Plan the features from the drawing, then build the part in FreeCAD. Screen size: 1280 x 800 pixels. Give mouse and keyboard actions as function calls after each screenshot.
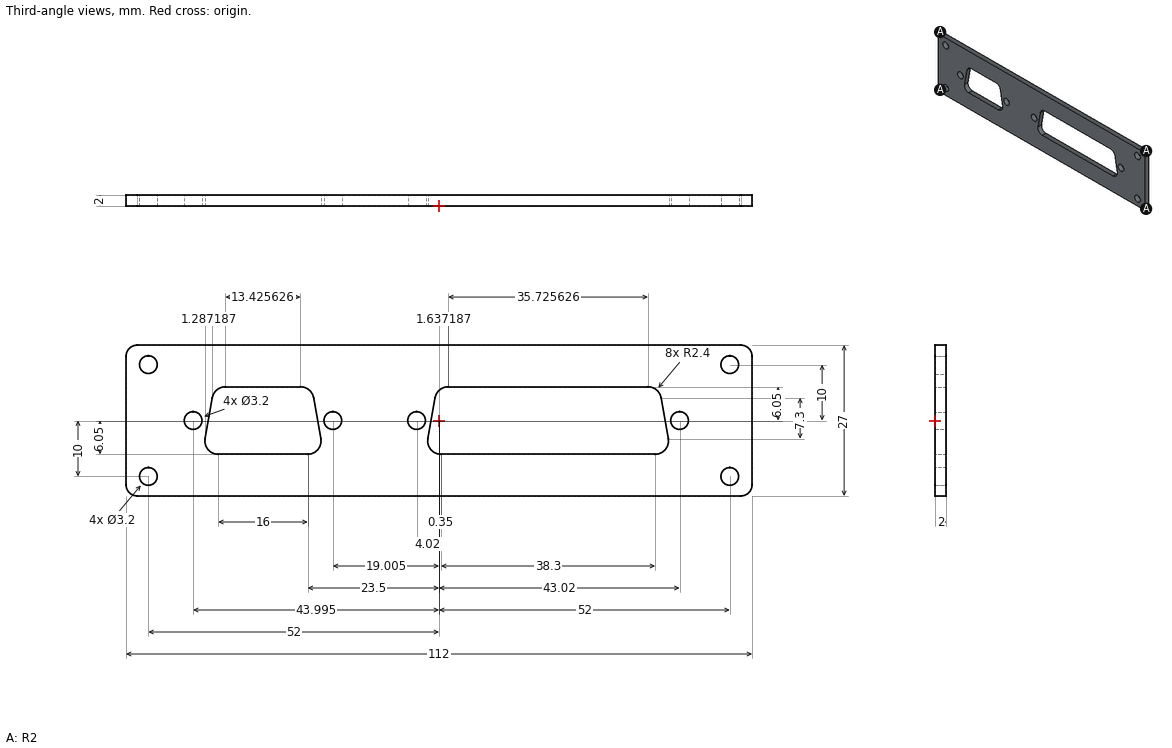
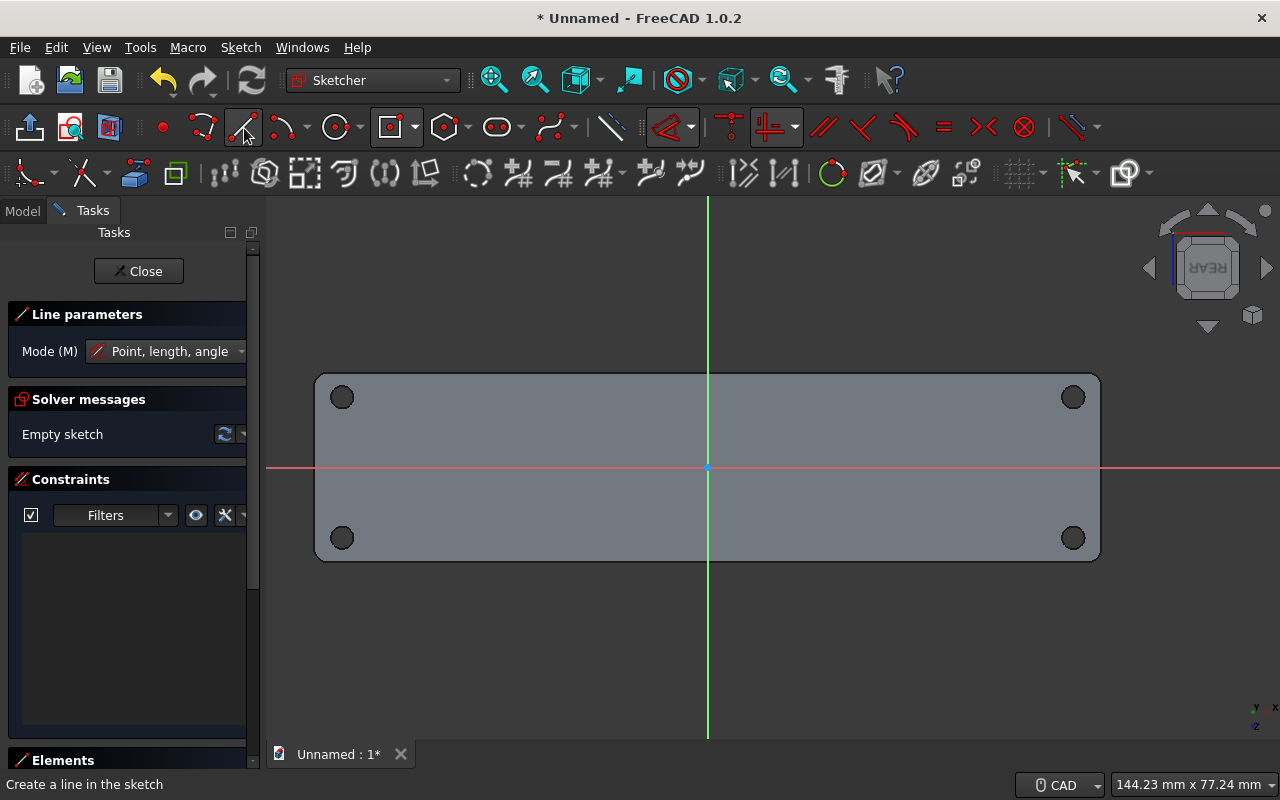
scroll(719, 510, up, 2)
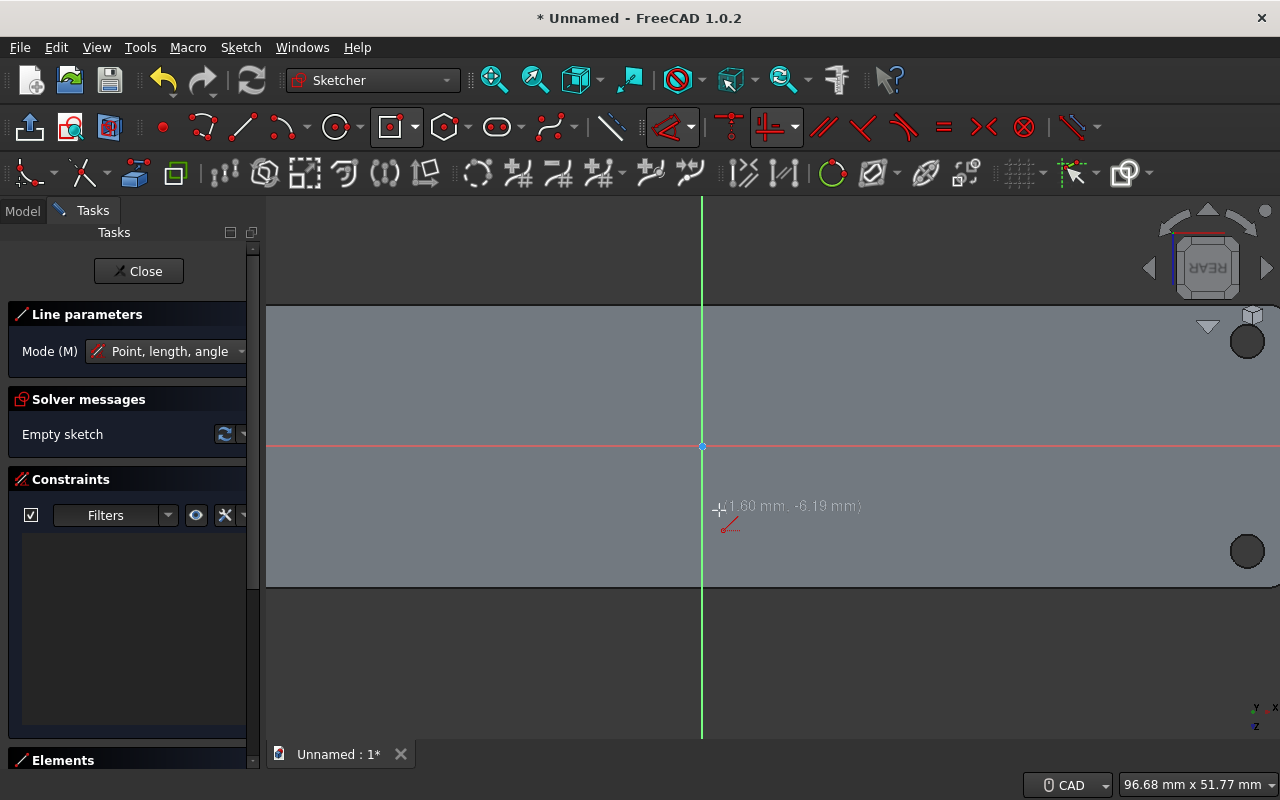
click(719, 510)
click(1094, 510)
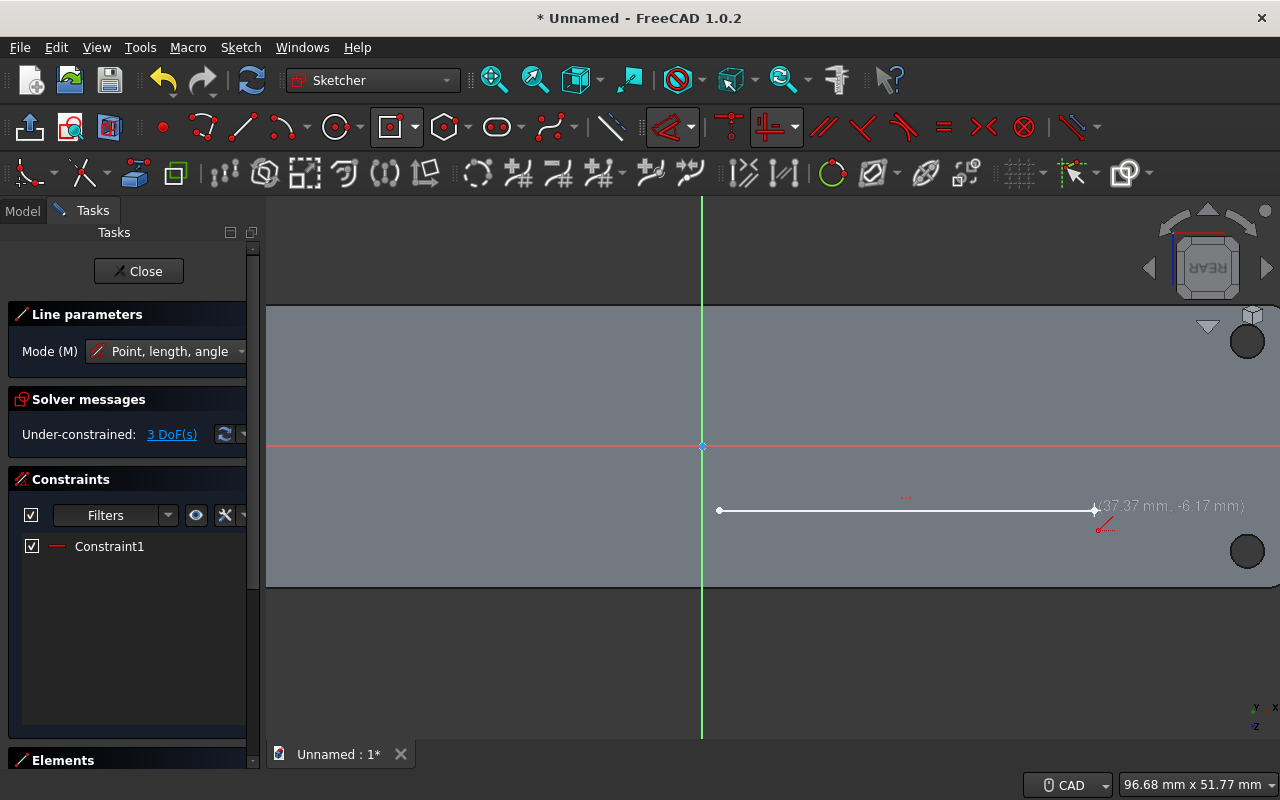
scroll(720, 511, down, 2)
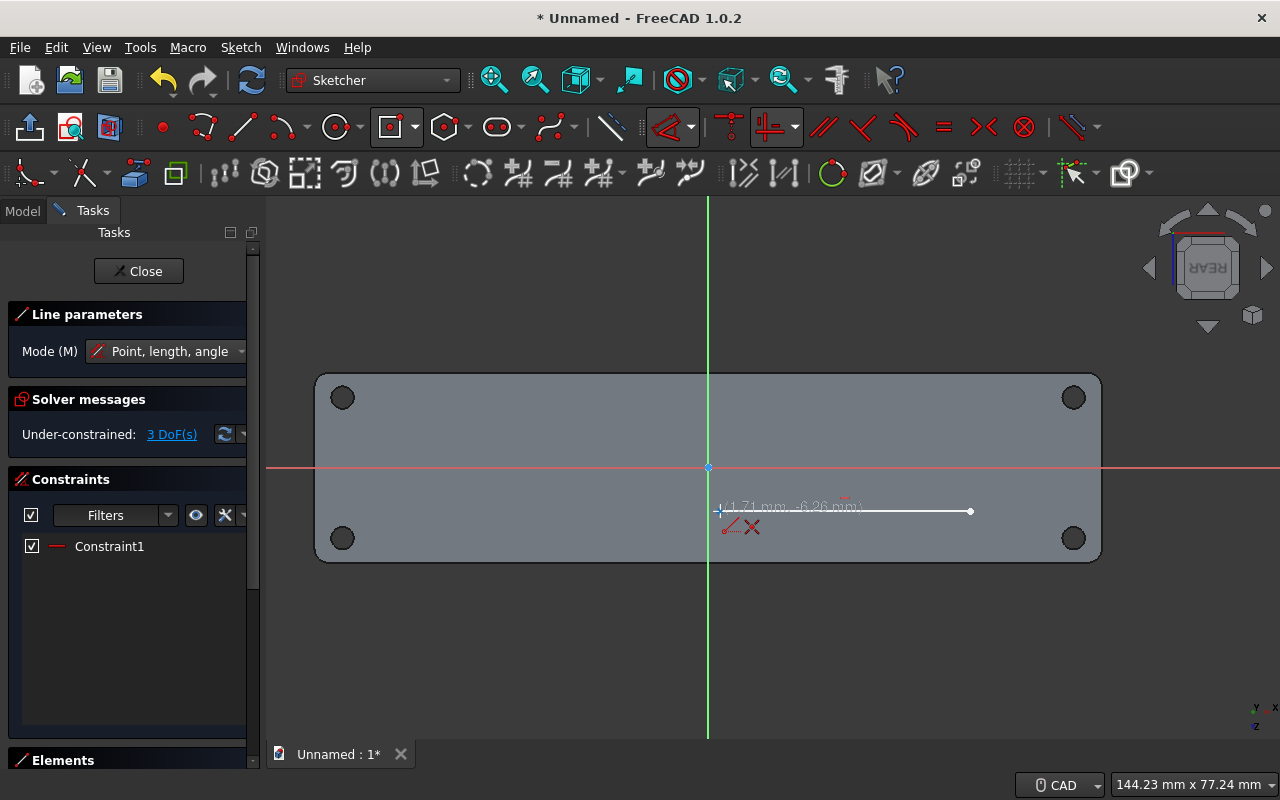
click(987, 496)
click(996, 445)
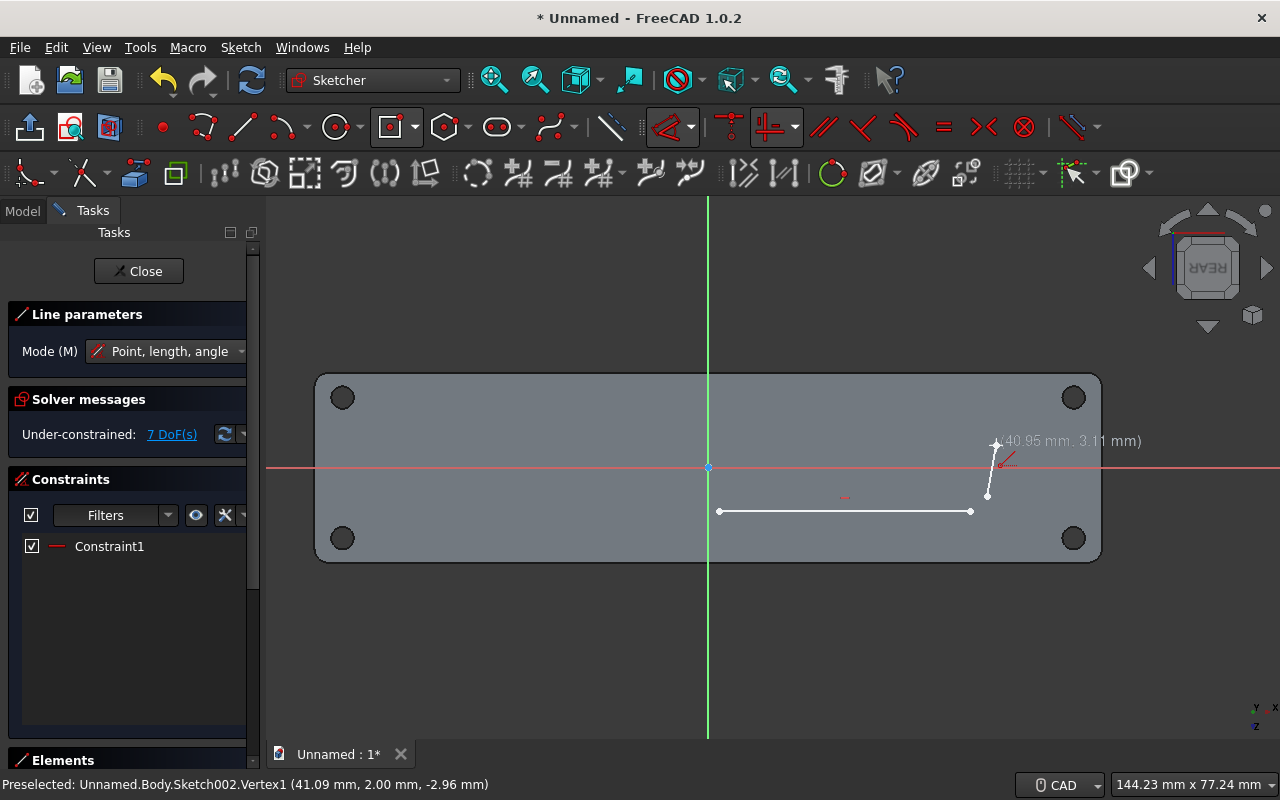
click(980, 425)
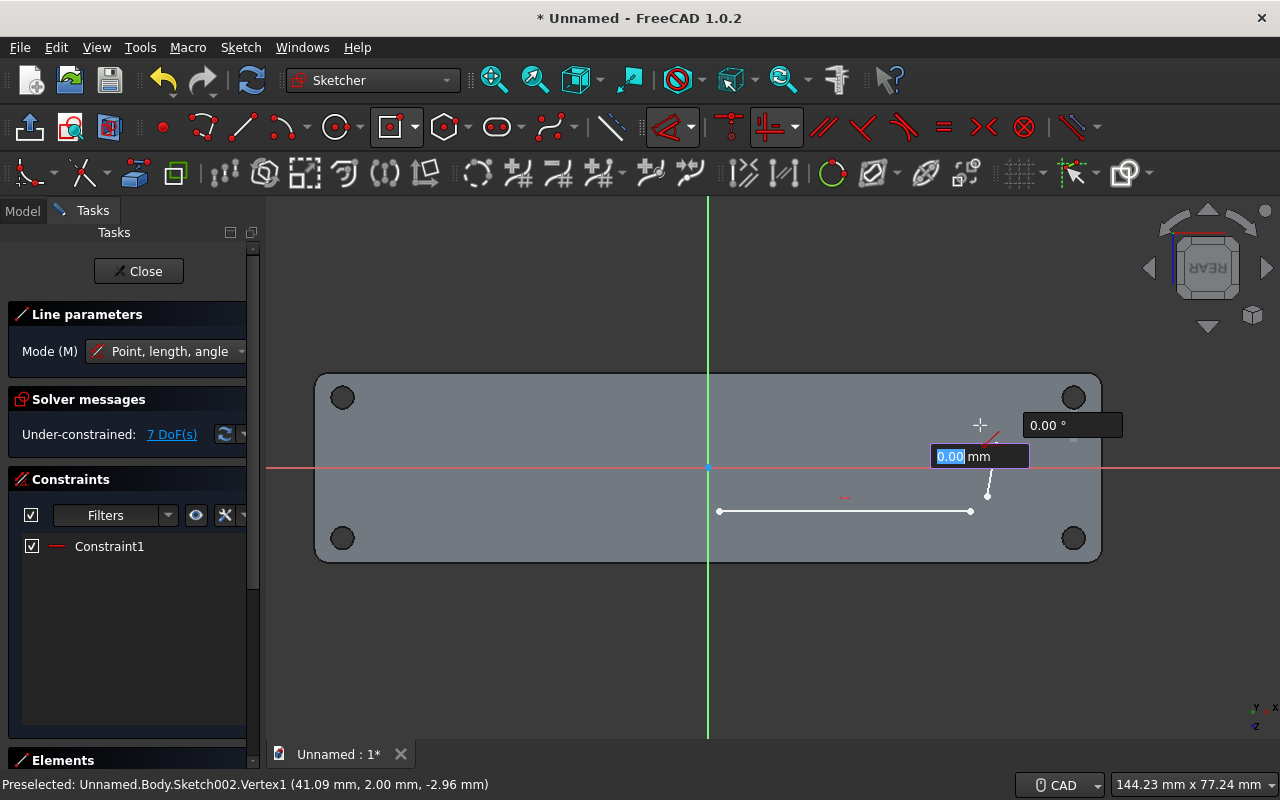
scroll(711, 425, up, 10)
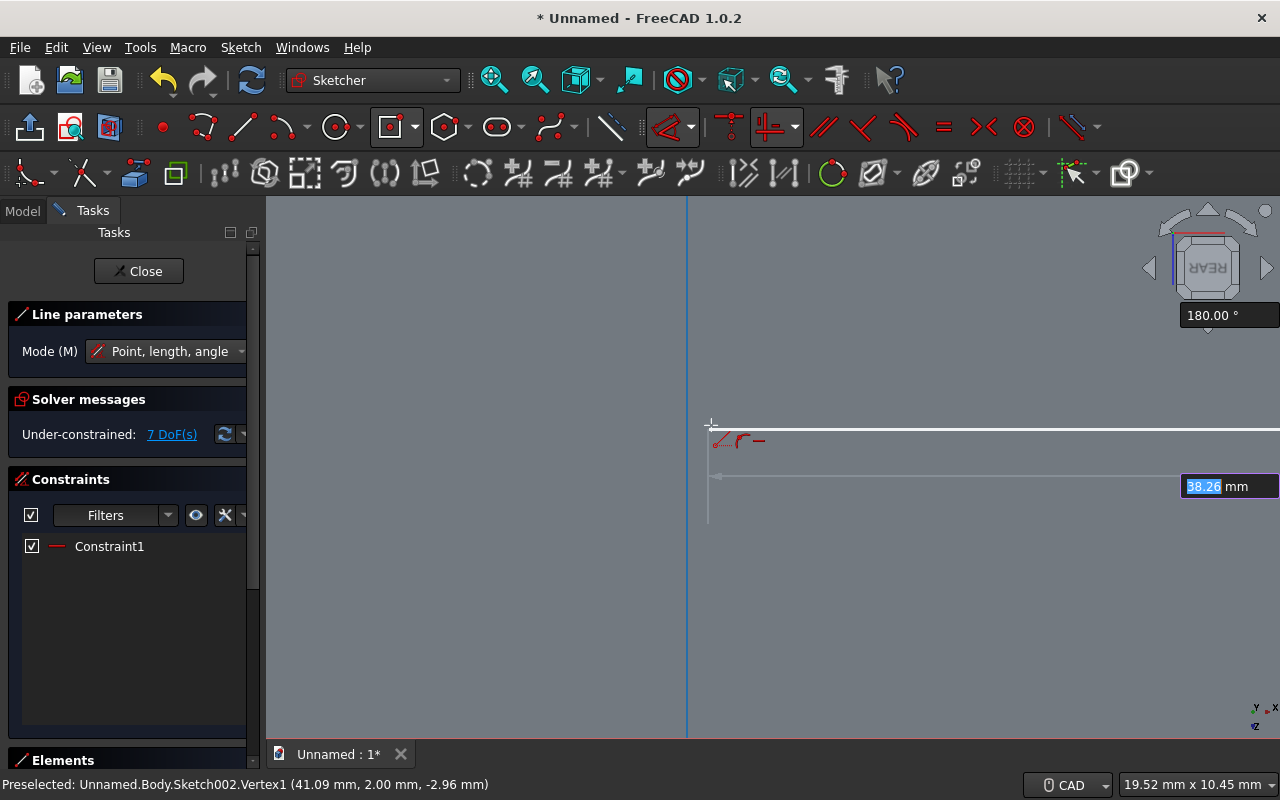
click(705, 422)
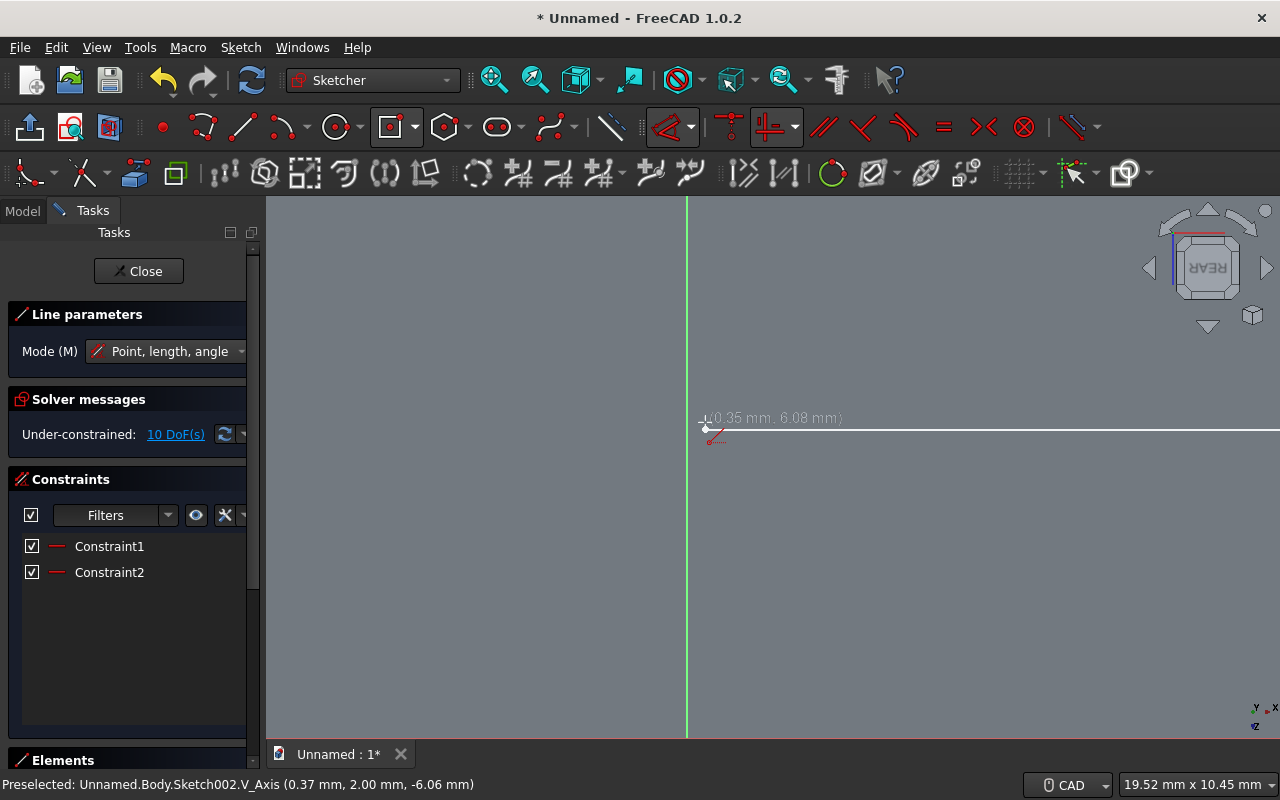
scroll(711, 425, down, 10)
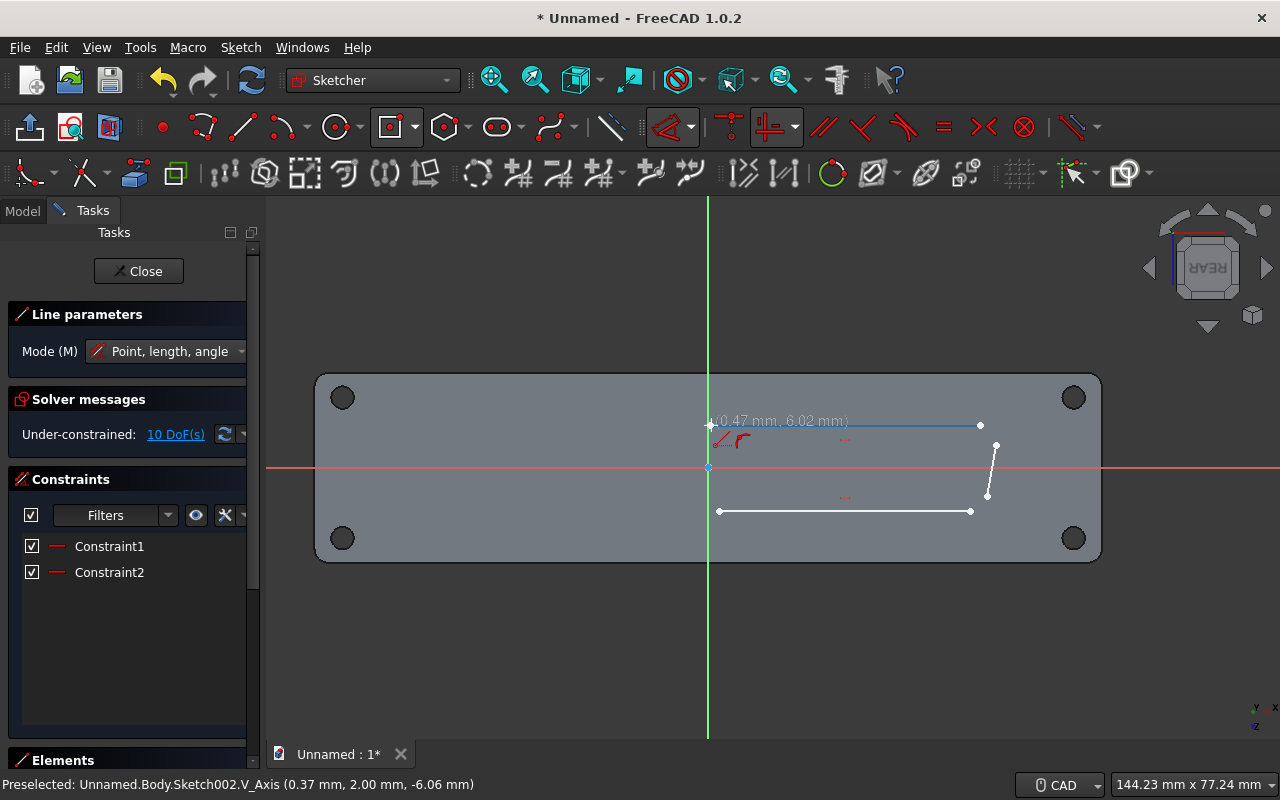
click(694, 445)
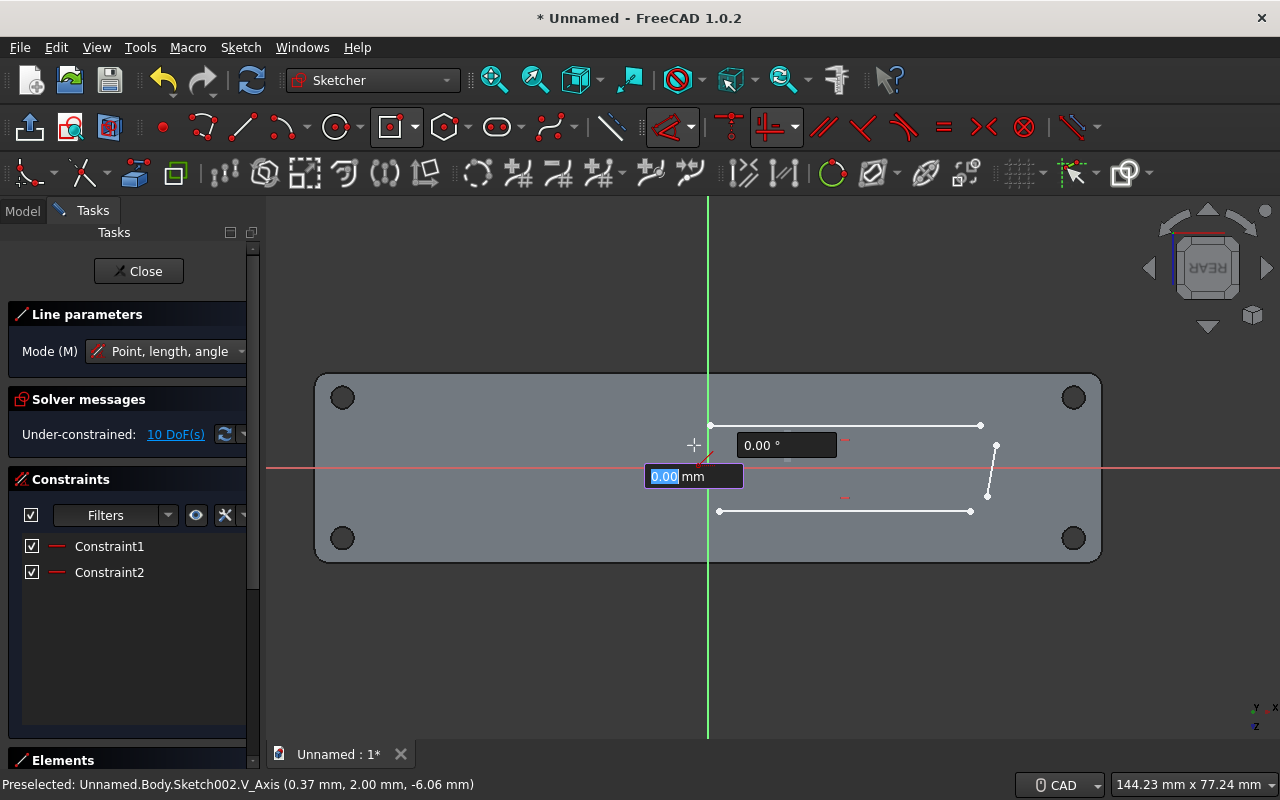
scroll(703, 496, up, 6)